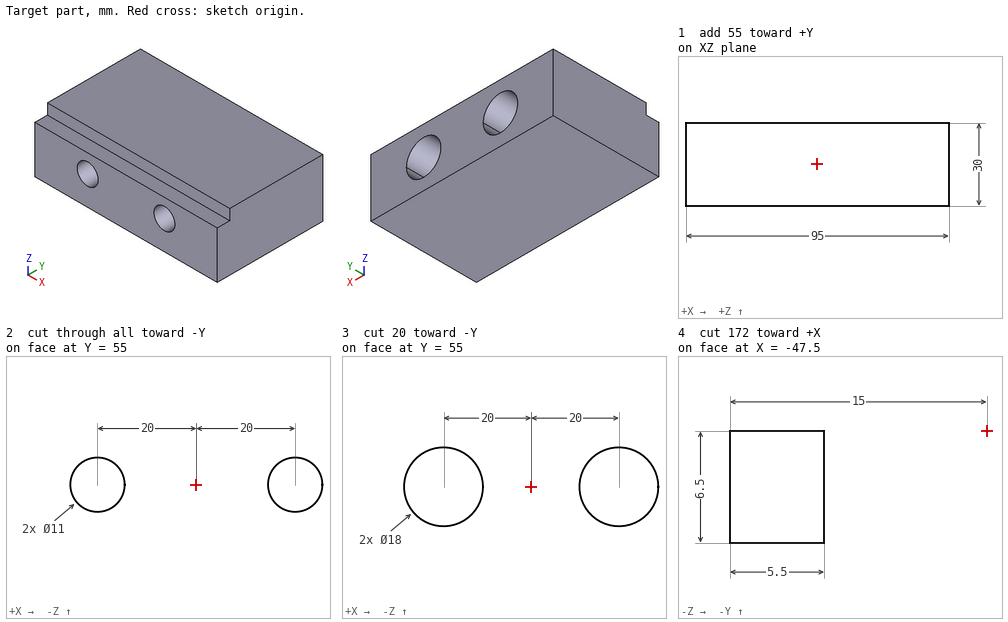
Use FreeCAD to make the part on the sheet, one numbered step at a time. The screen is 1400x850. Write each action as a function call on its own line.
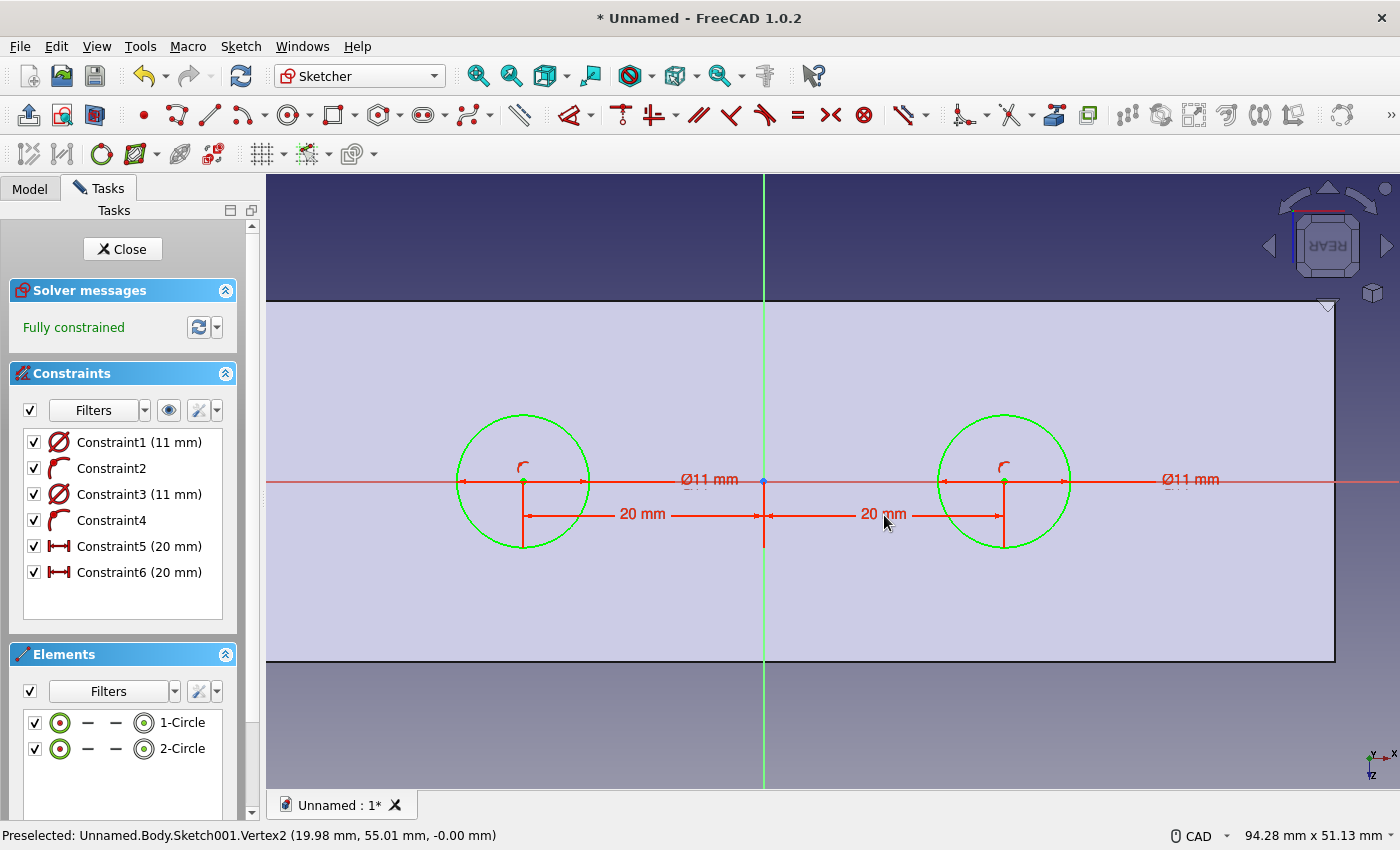
click(123, 249)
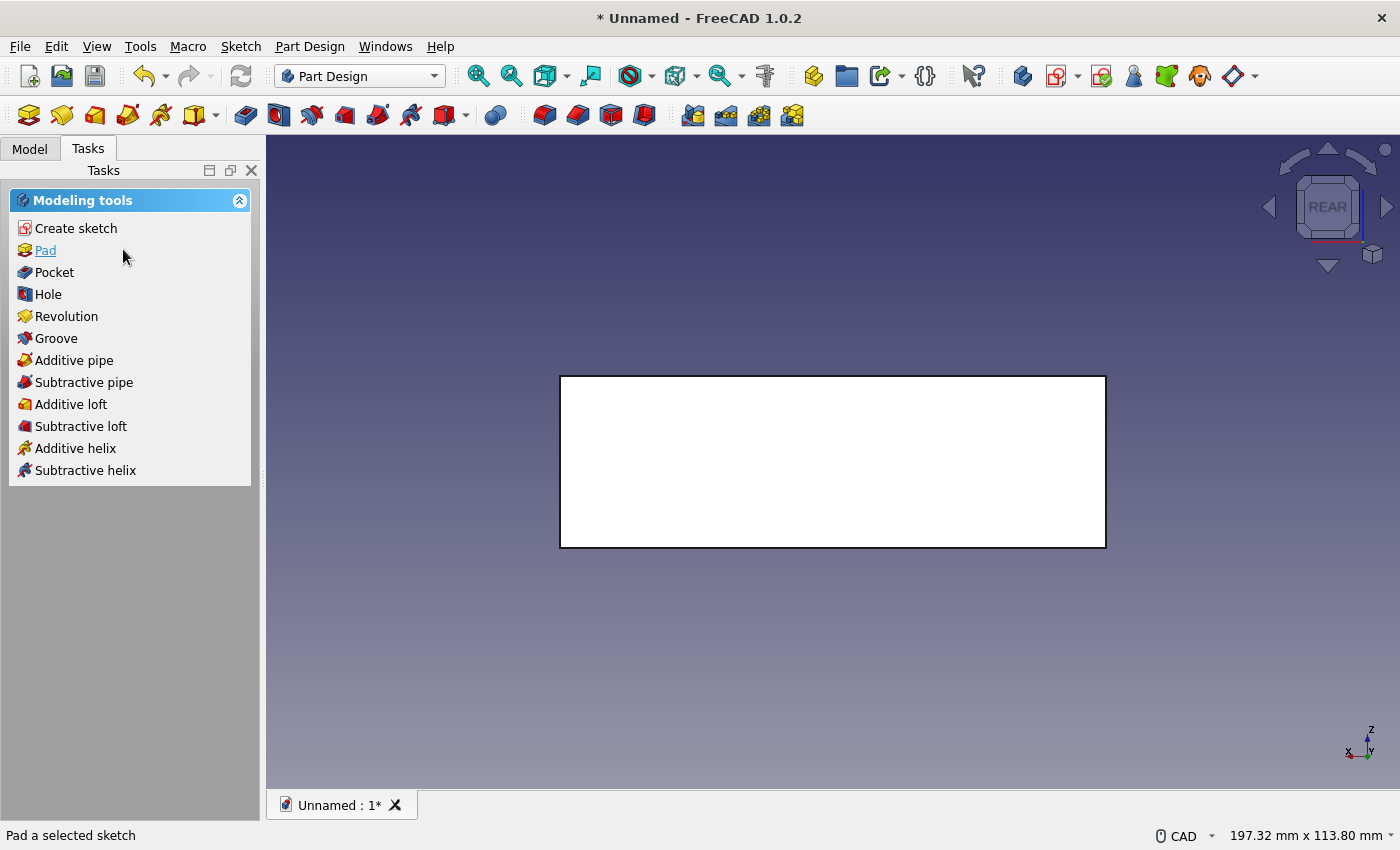
click(246, 116)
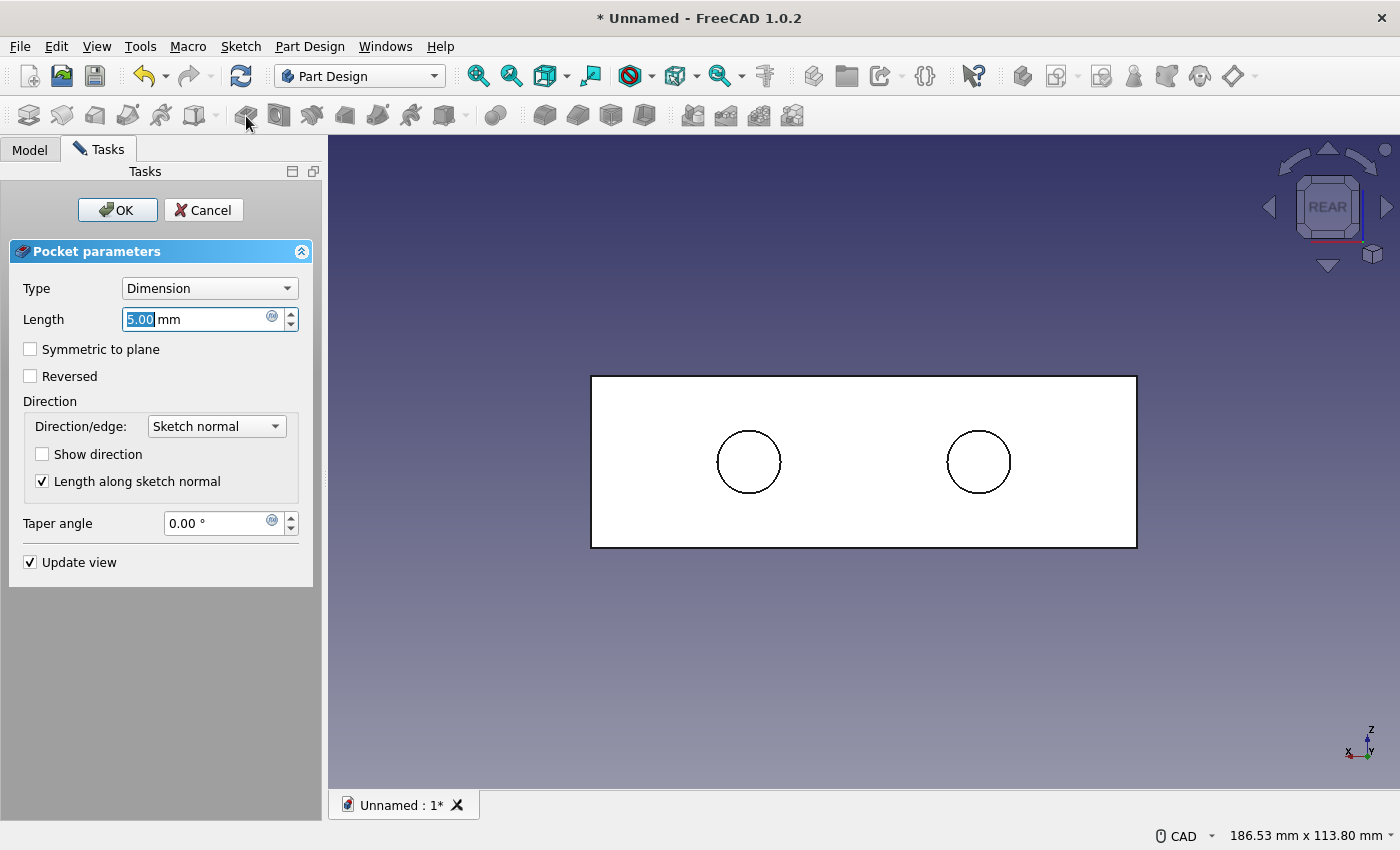
click(210, 288)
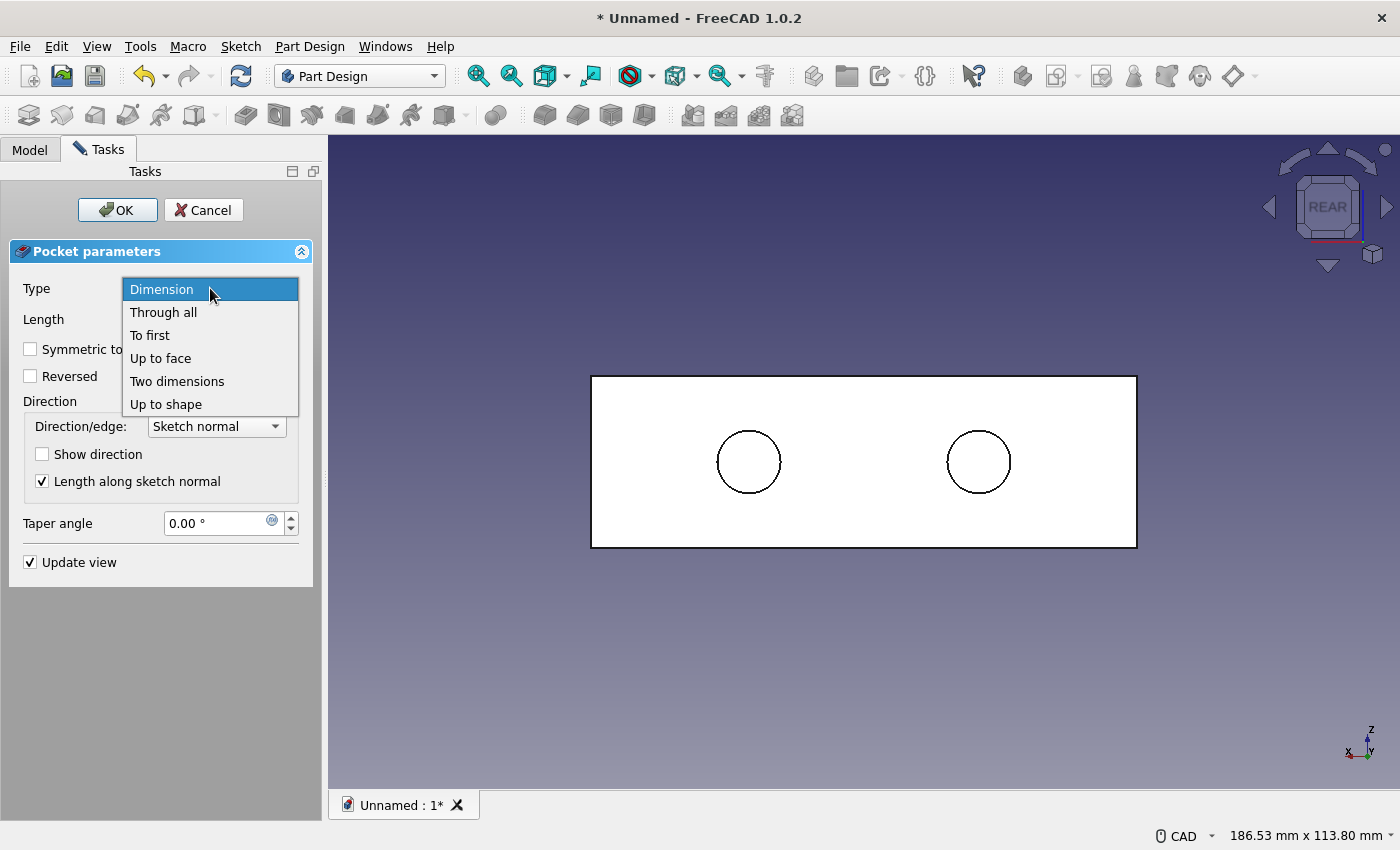
click(208, 312)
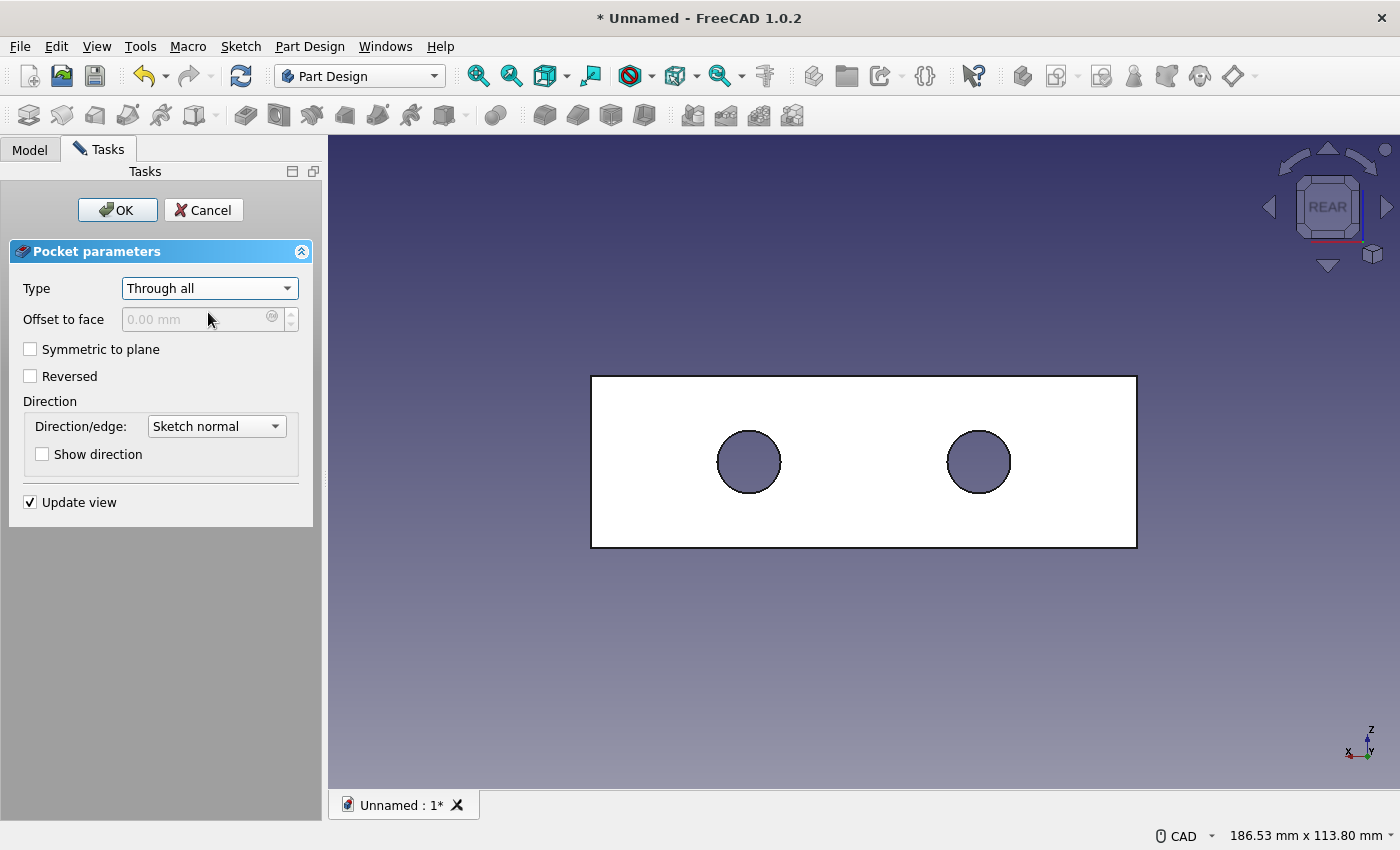
click(118, 210)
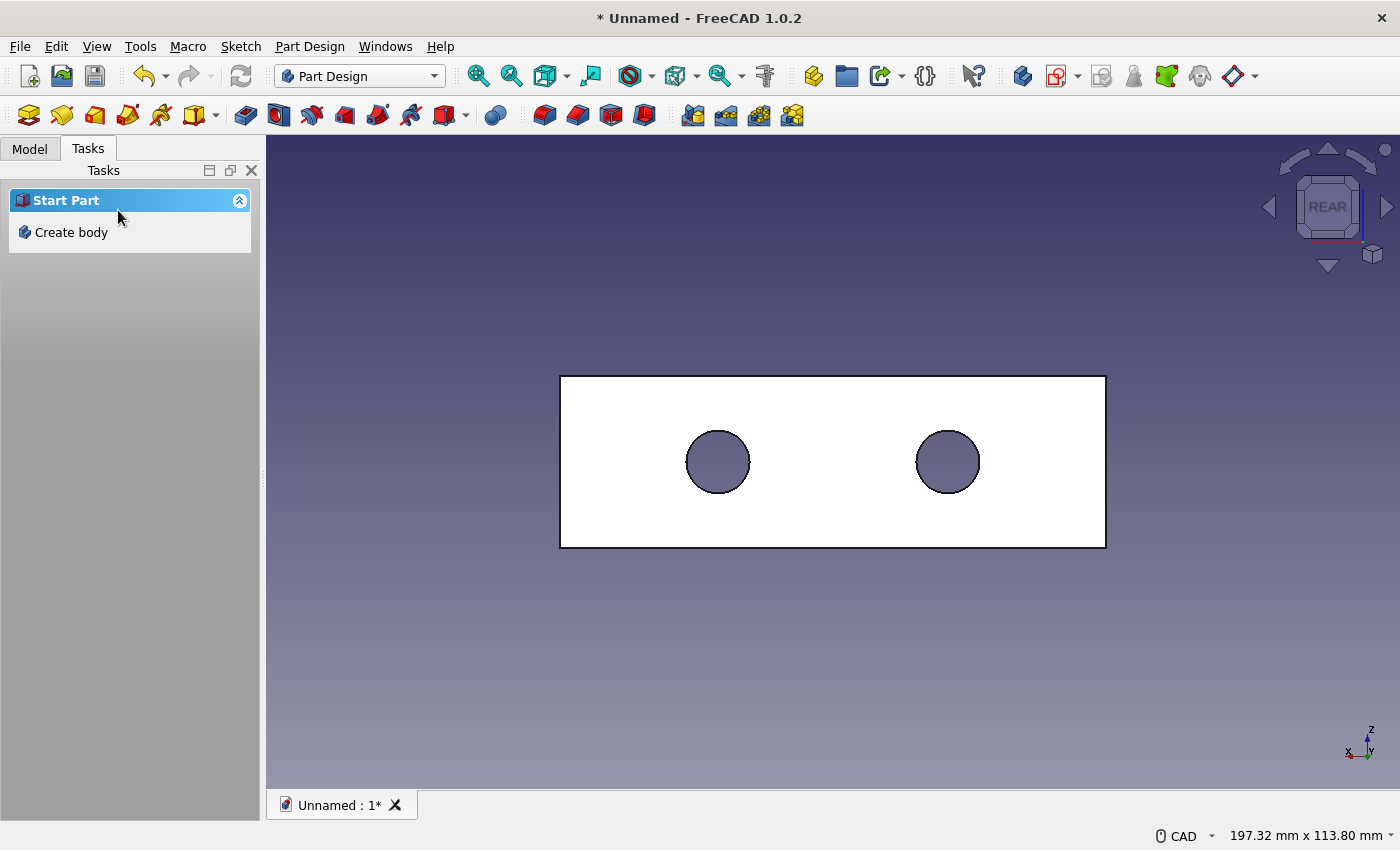
click(833, 461)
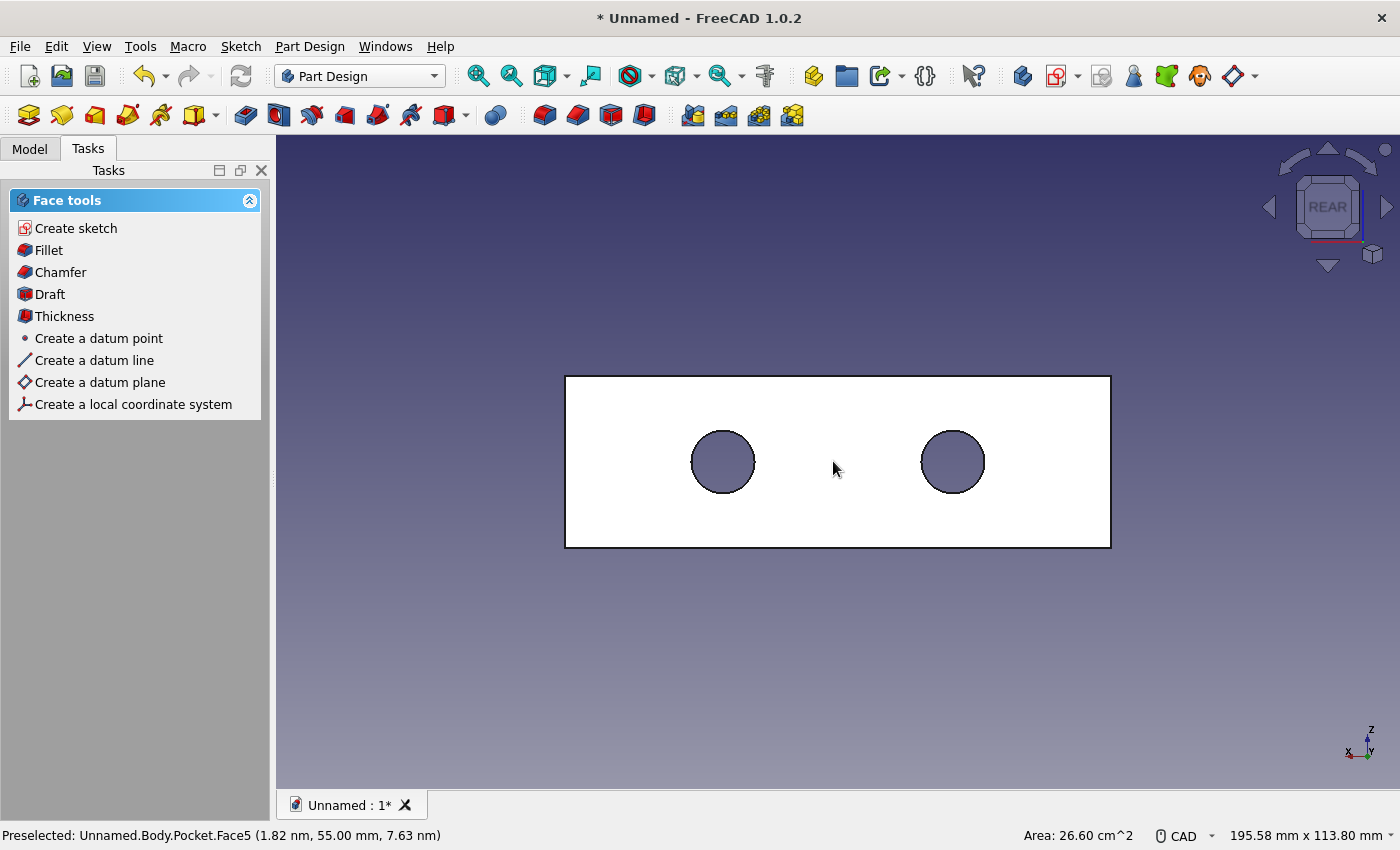
click(1056, 76)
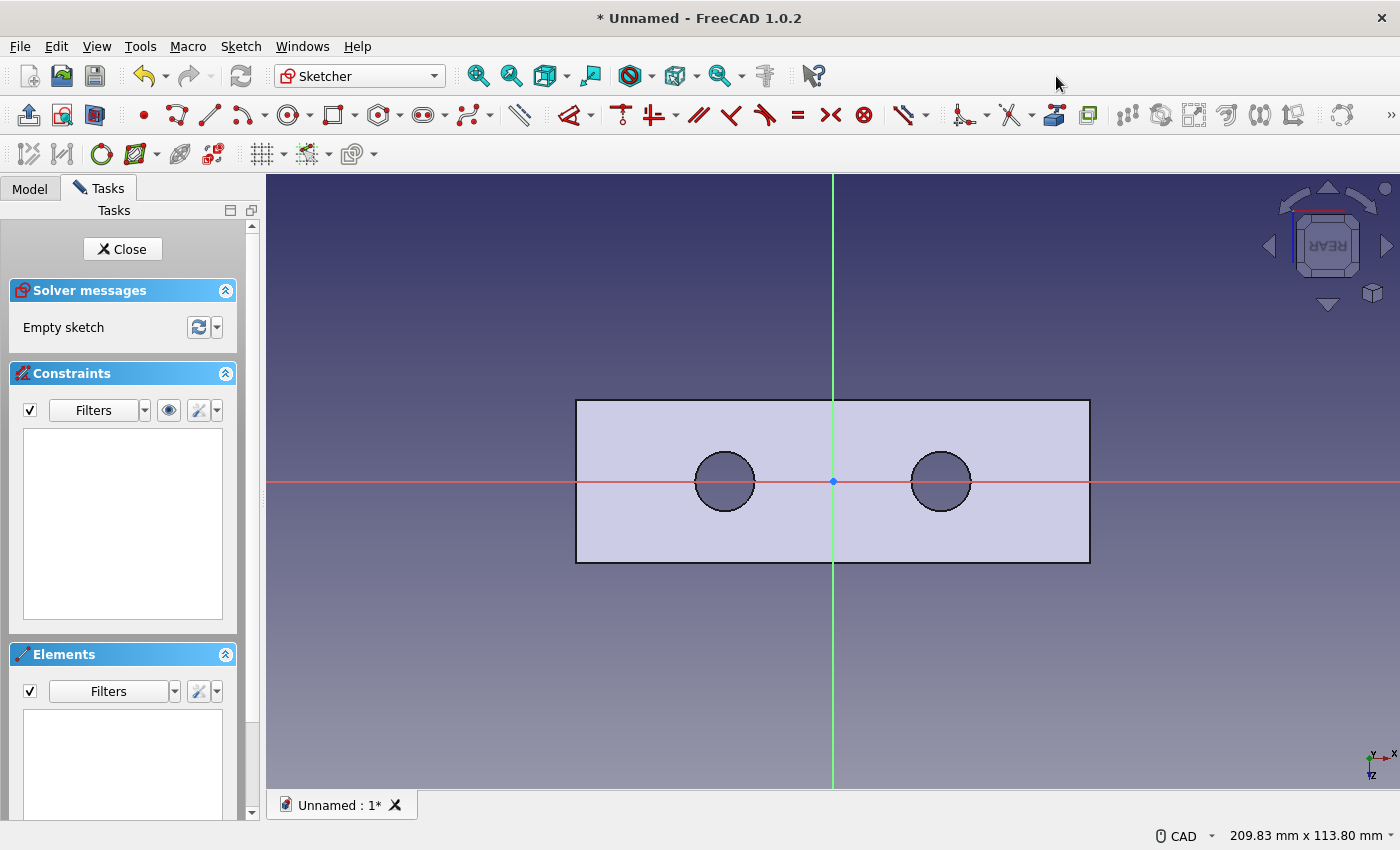
scroll(889, 481, up, 4)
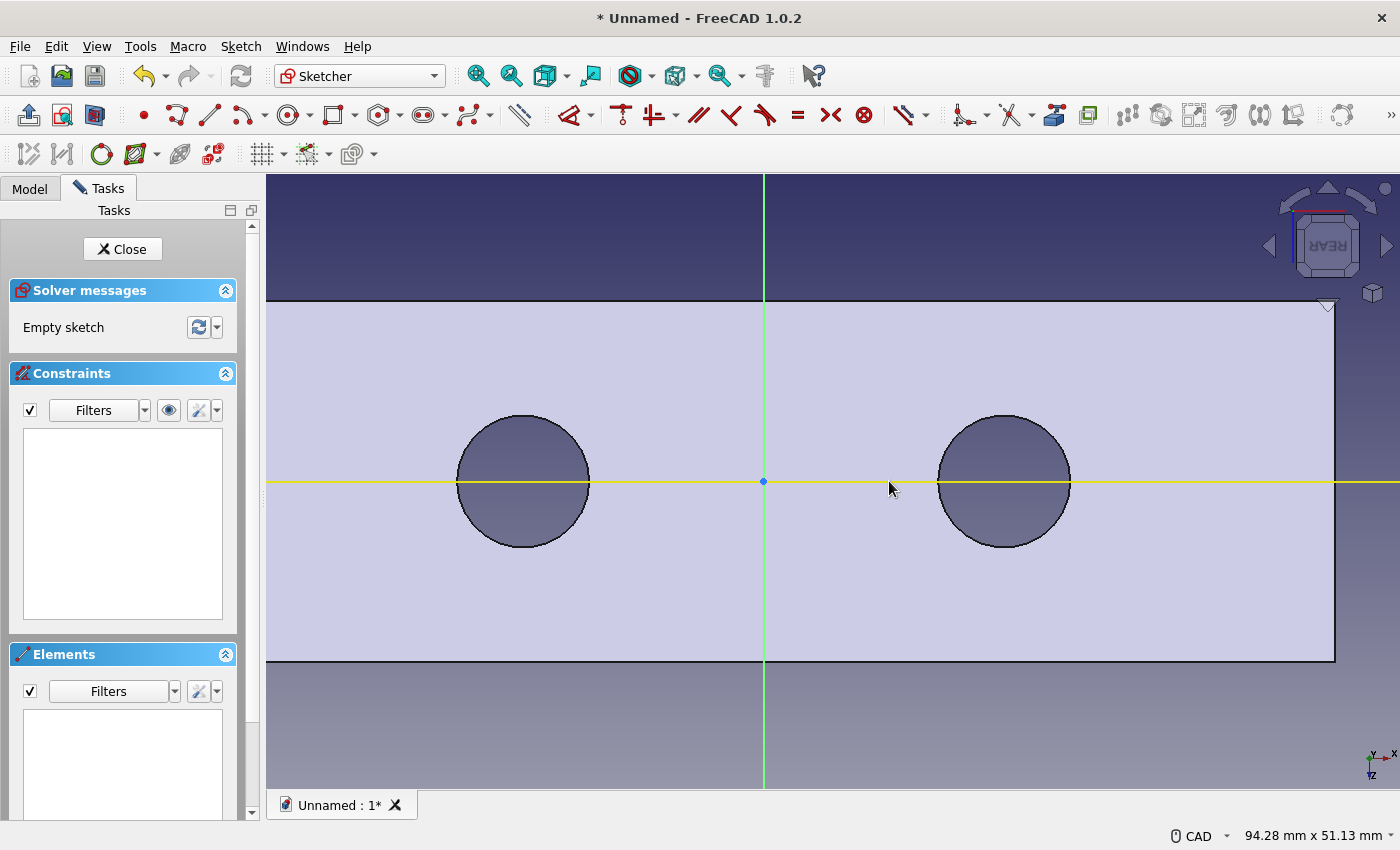
click(288, 116)